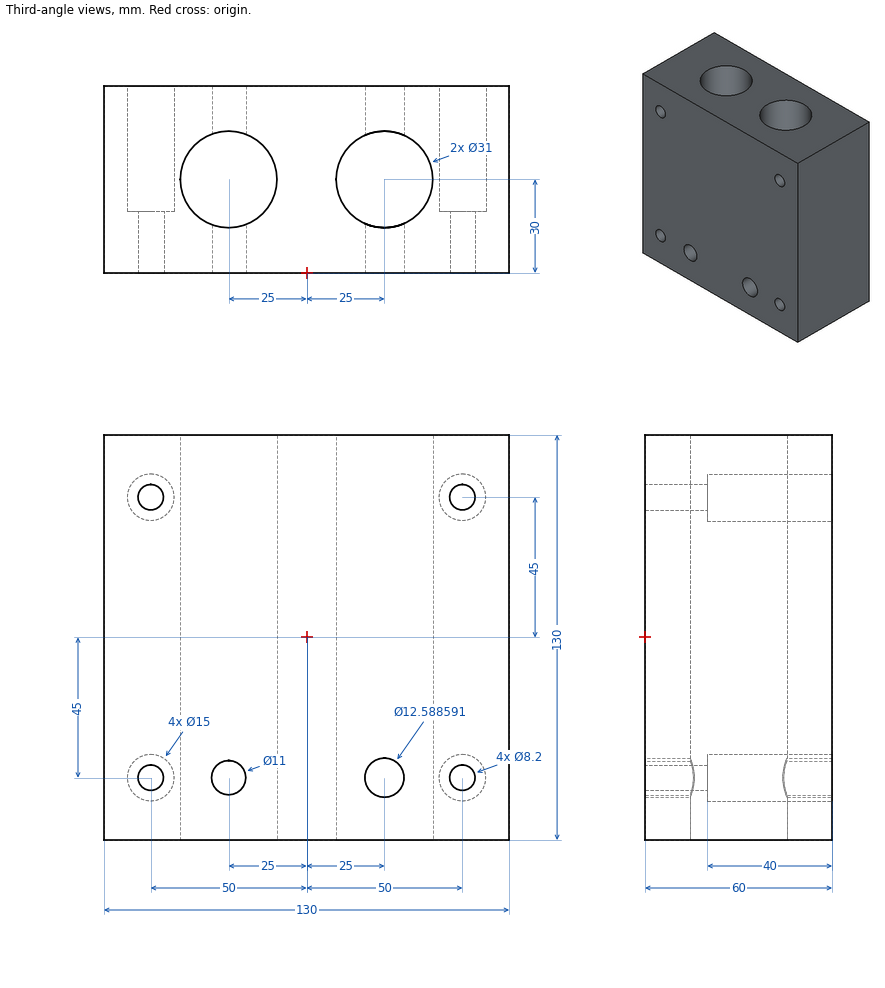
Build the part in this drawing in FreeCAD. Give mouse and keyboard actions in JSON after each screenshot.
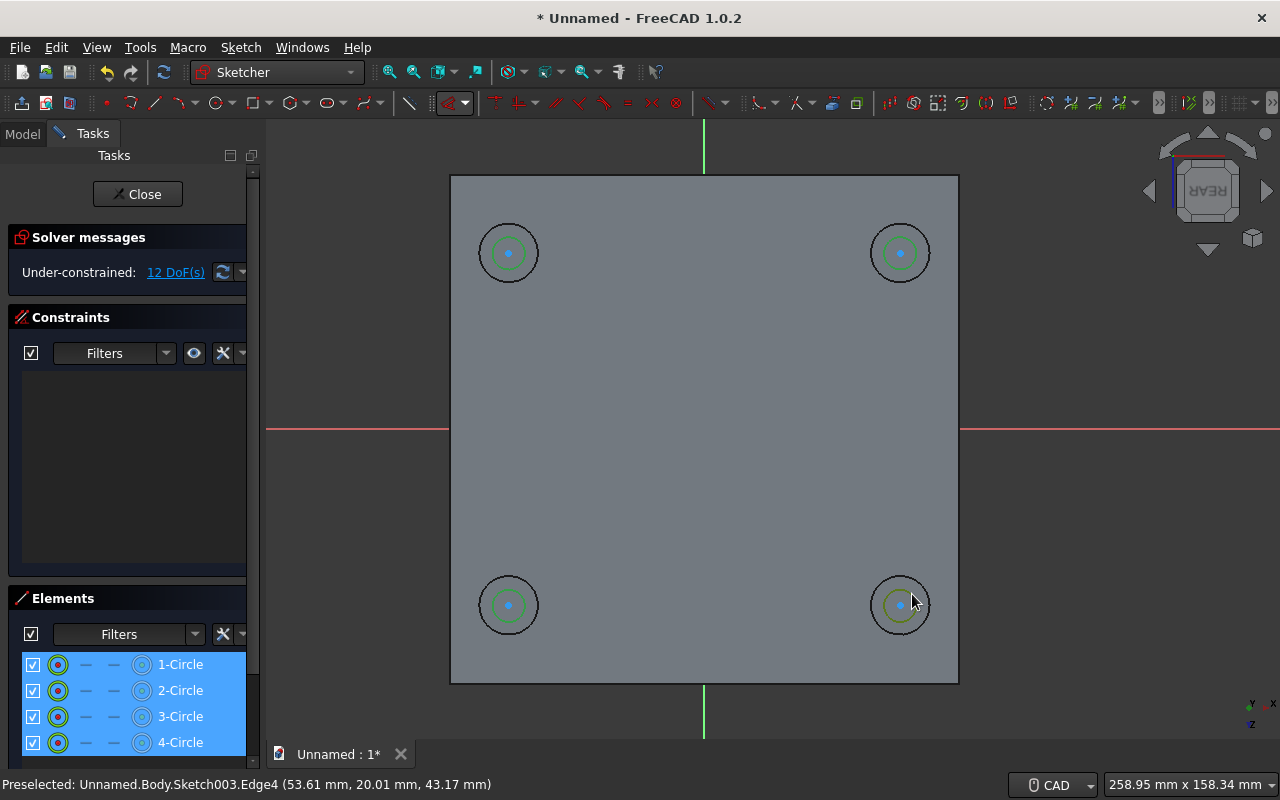
{"action": "key", "text": "e"}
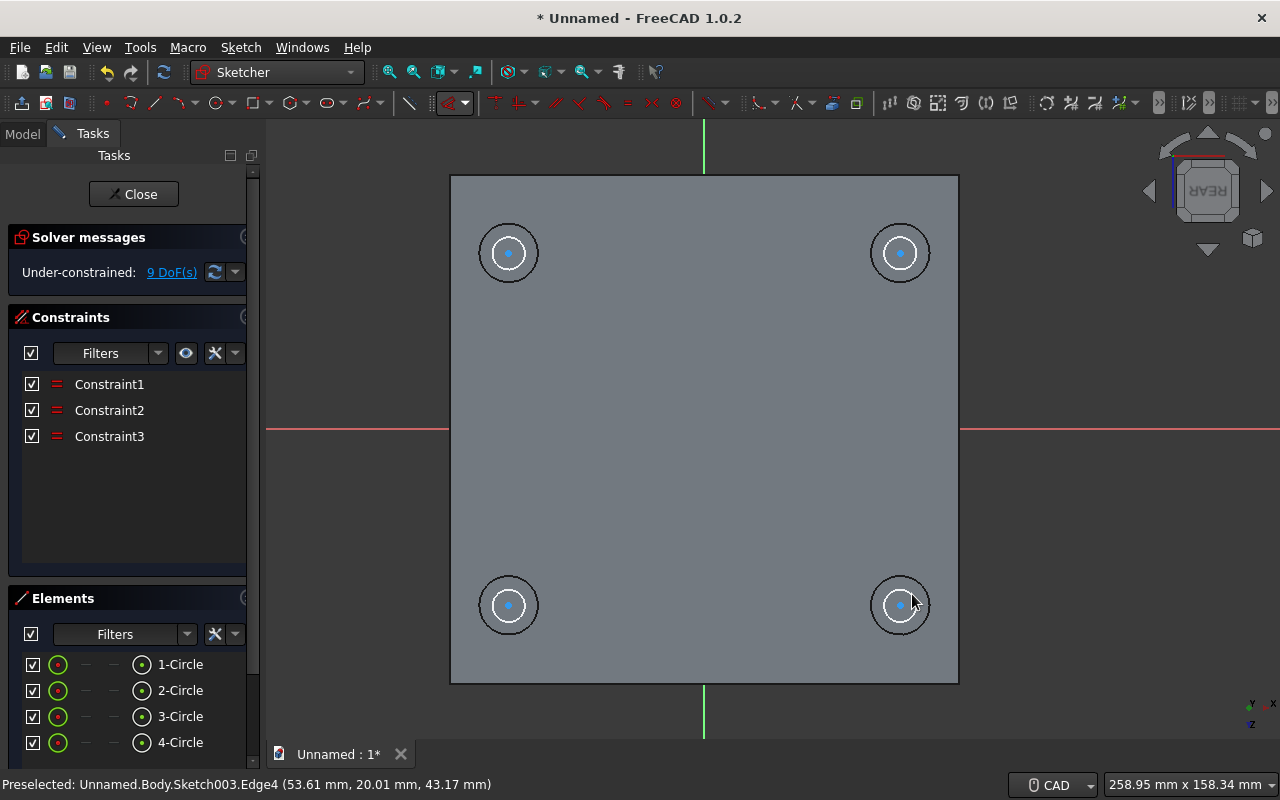
{"action": "left_click", "coordinate": [900, 253]}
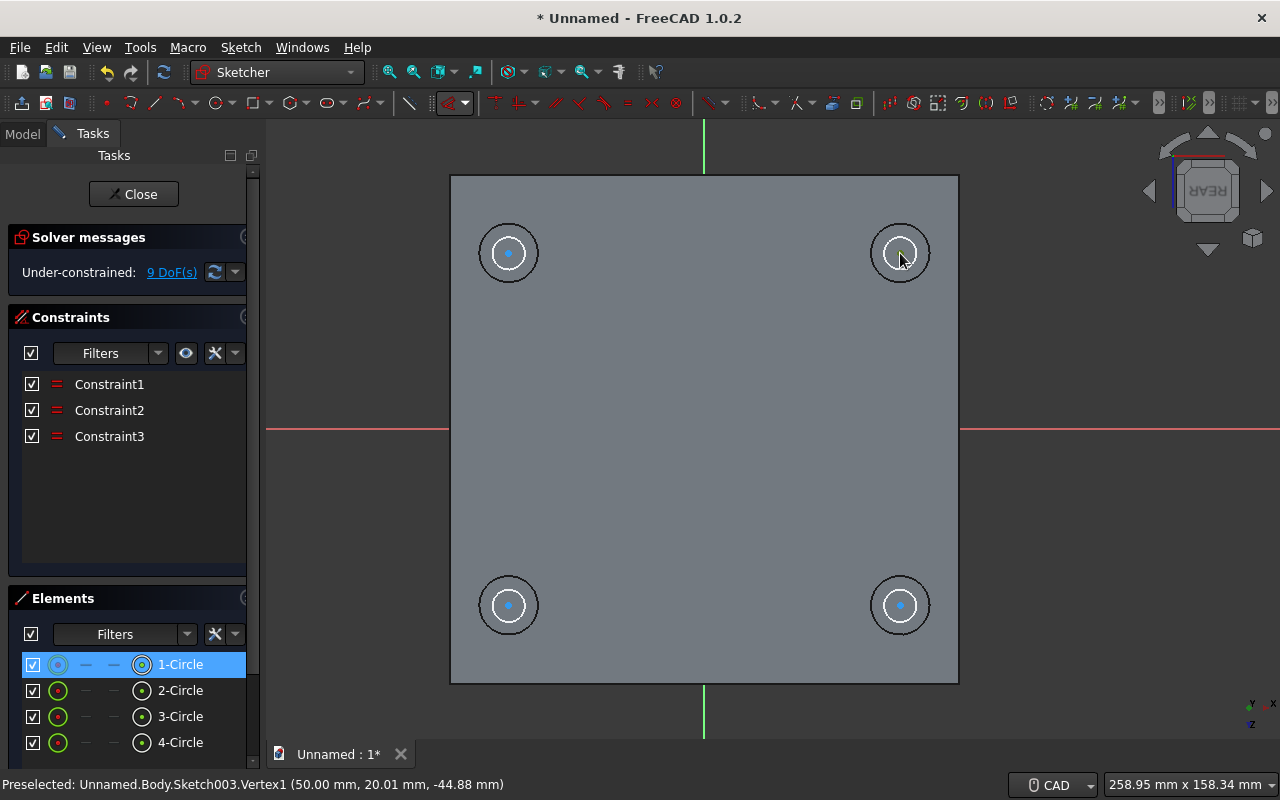
{"action": "left_click", "coordinate": [509, 253]}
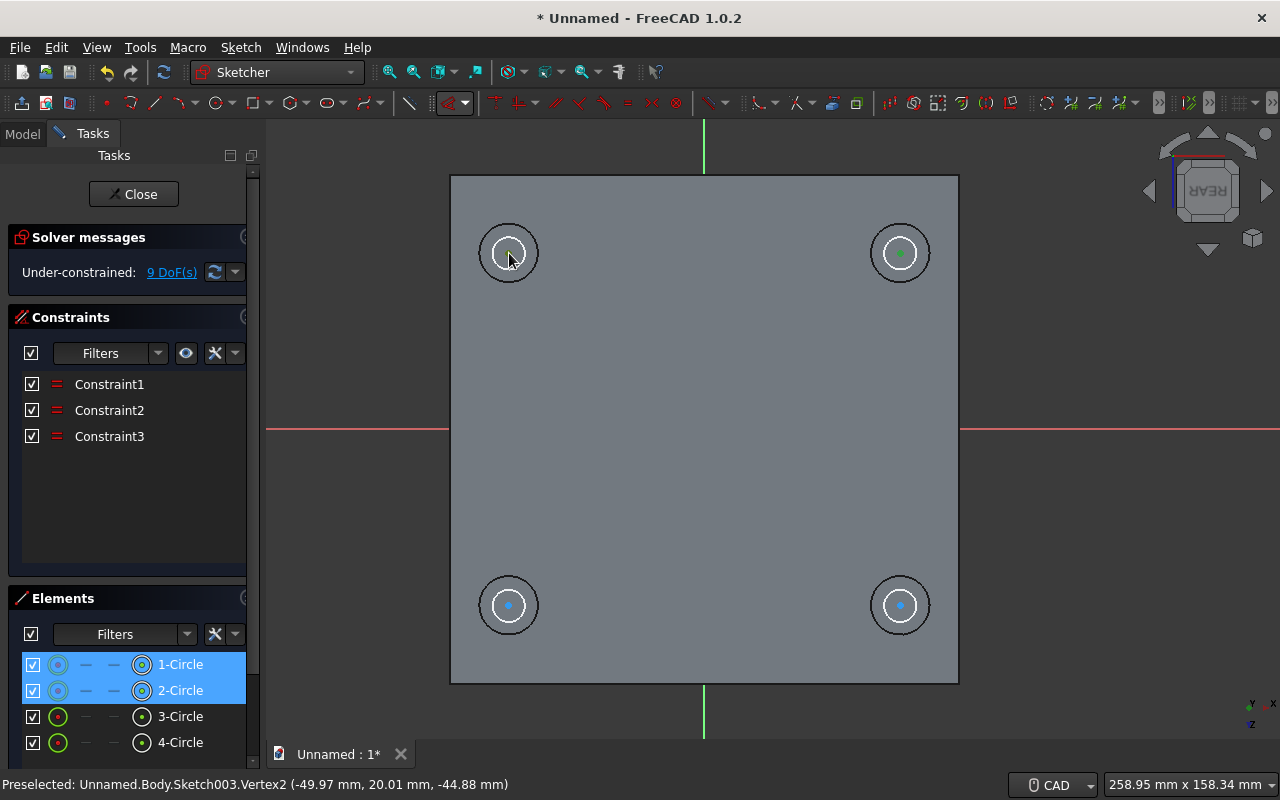
{"action": "key", "text": "h"}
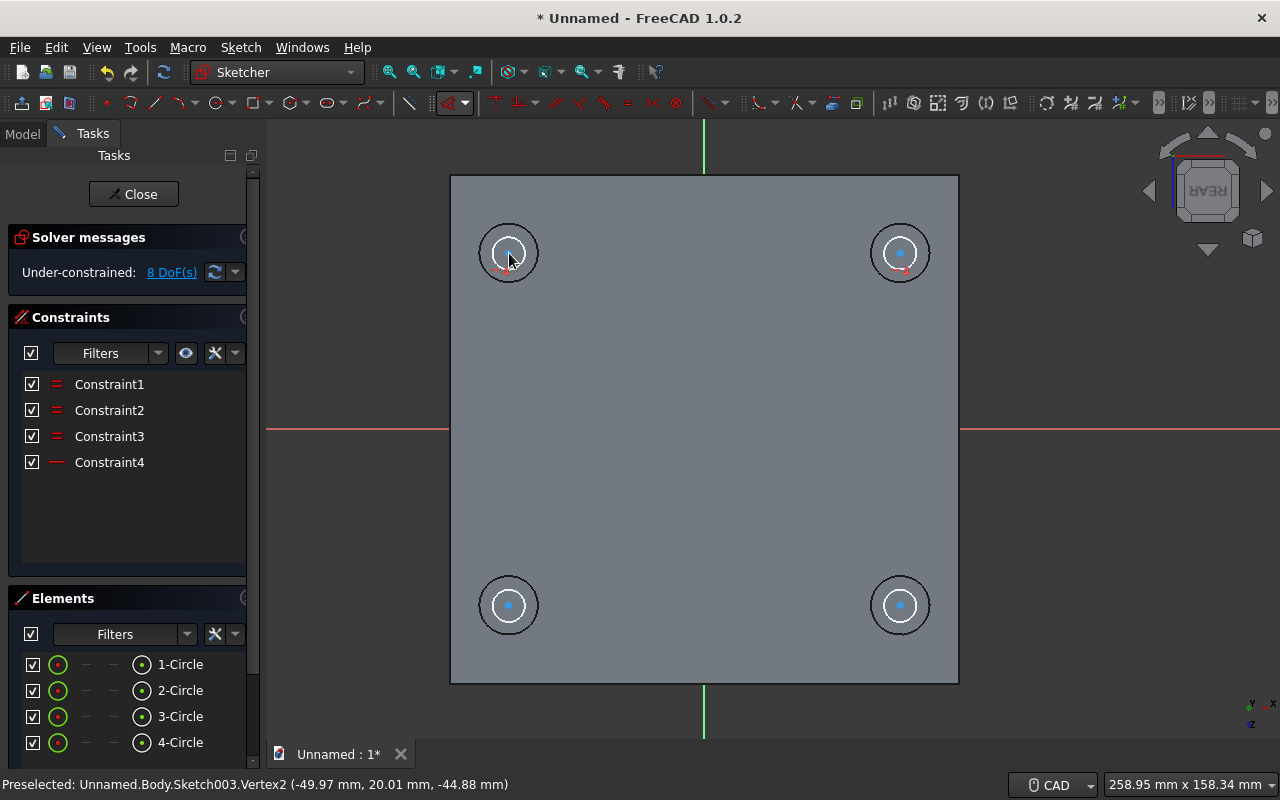
{"action": "left_click", "coordinate": [509, 253]}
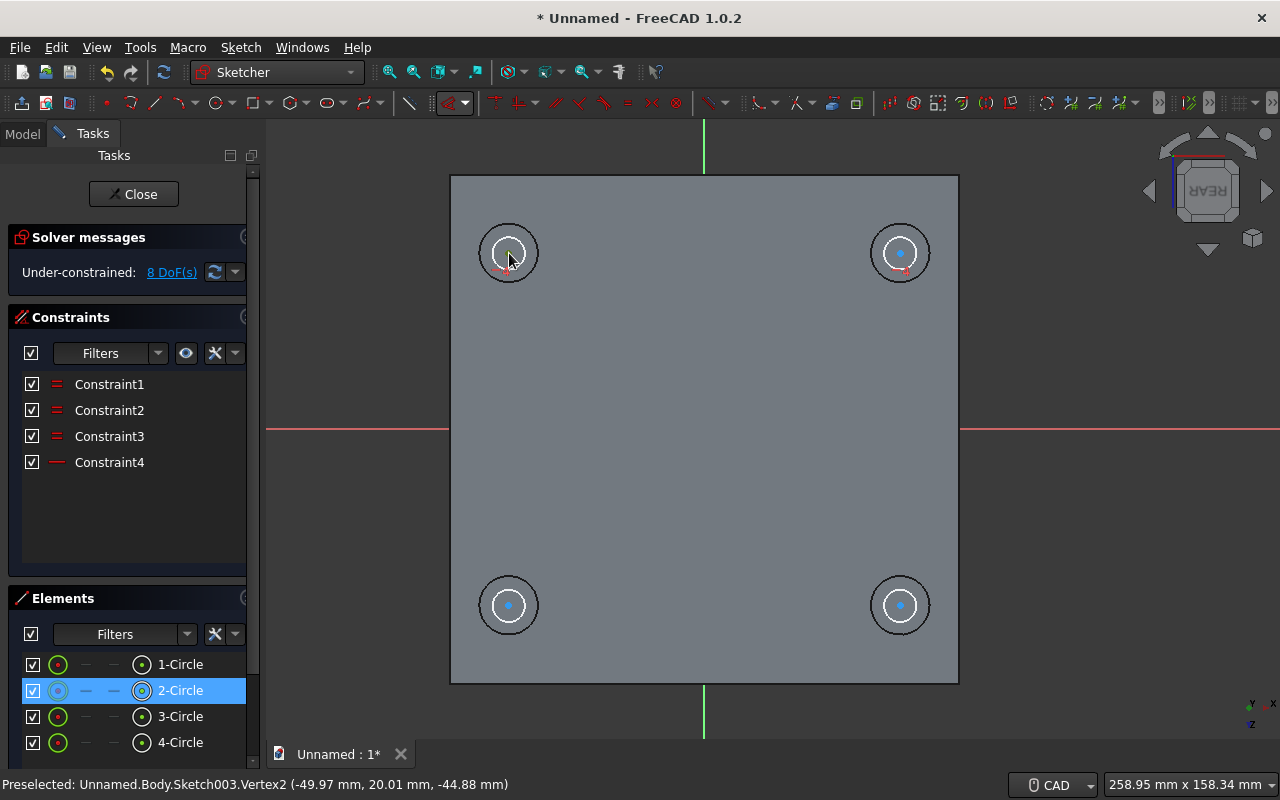
{"action": "left_click", "coordinate": [509, 606]}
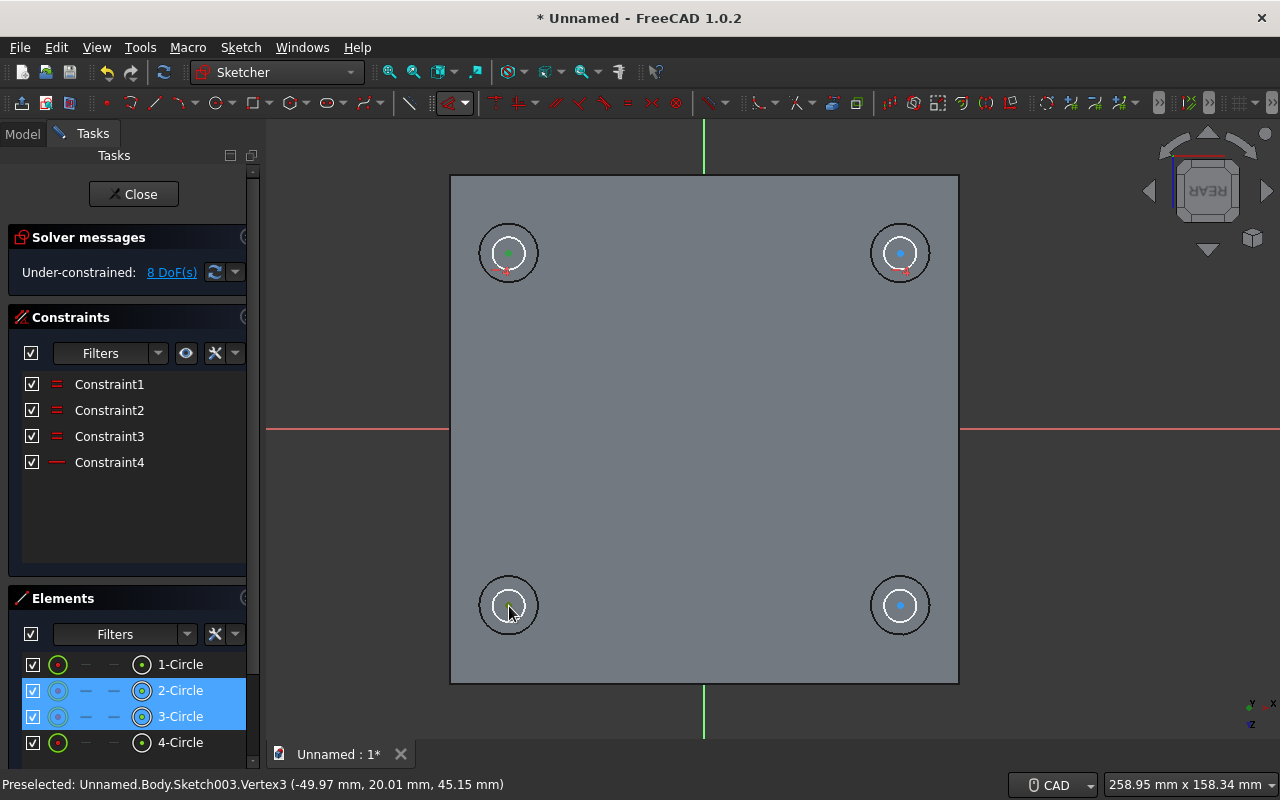
{"action": "key", "text": "v"}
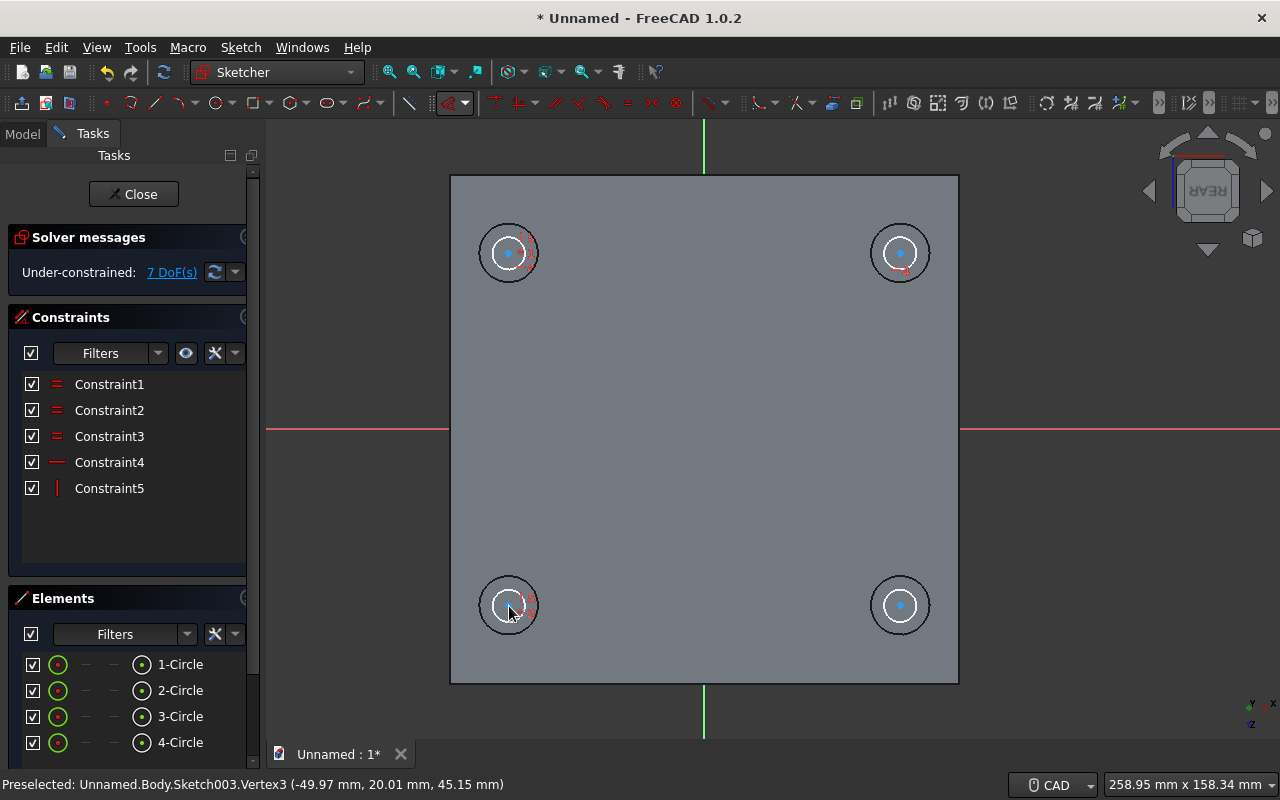
{"action": "left_click", "coordinate": [900, 253]}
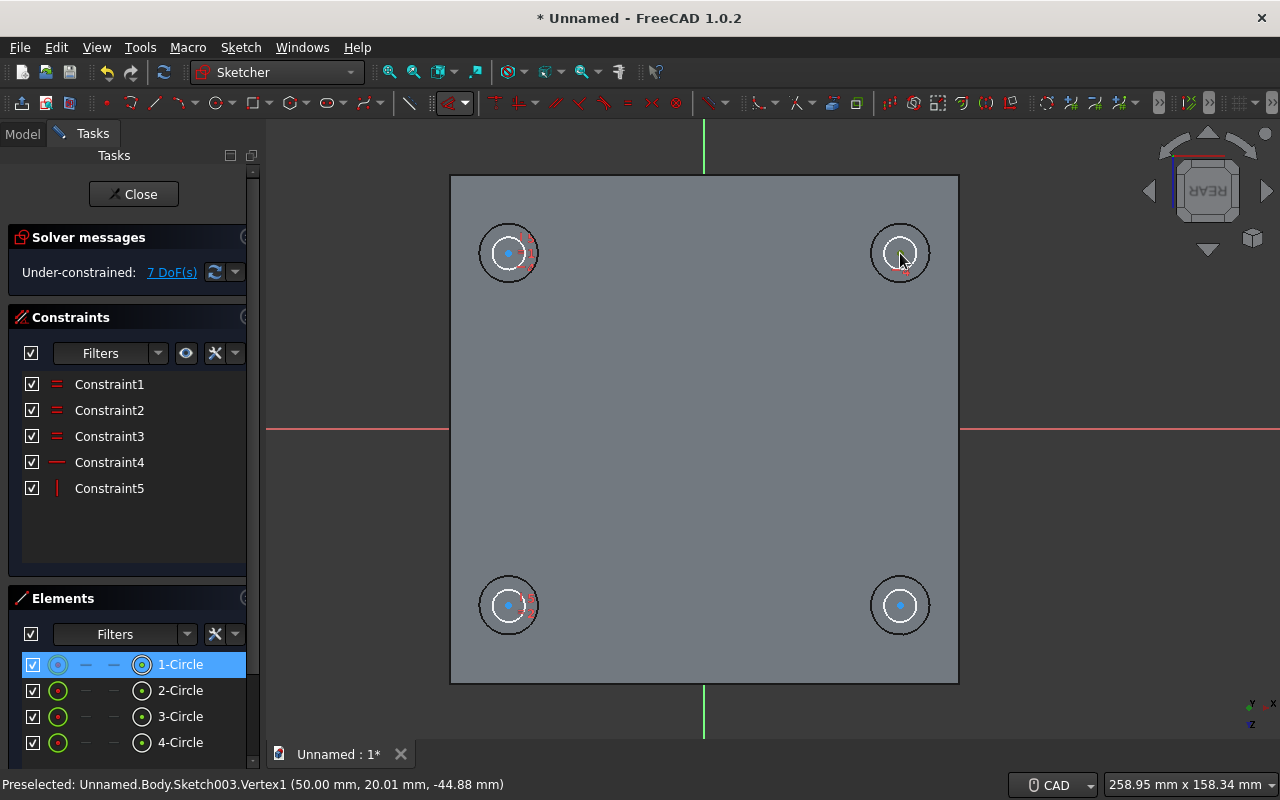
{"action": "left_click", "coordinate": [900, 606]}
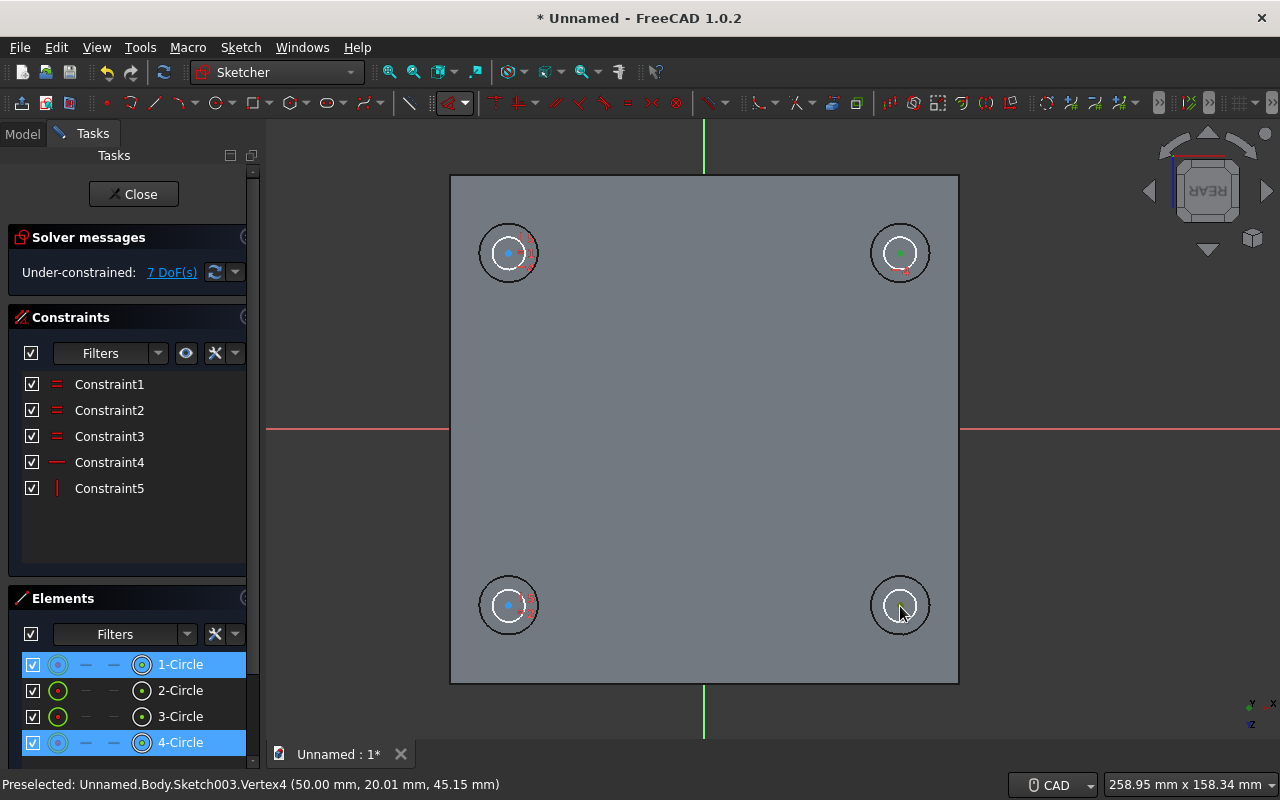
{"action": "key", "text": "v"}